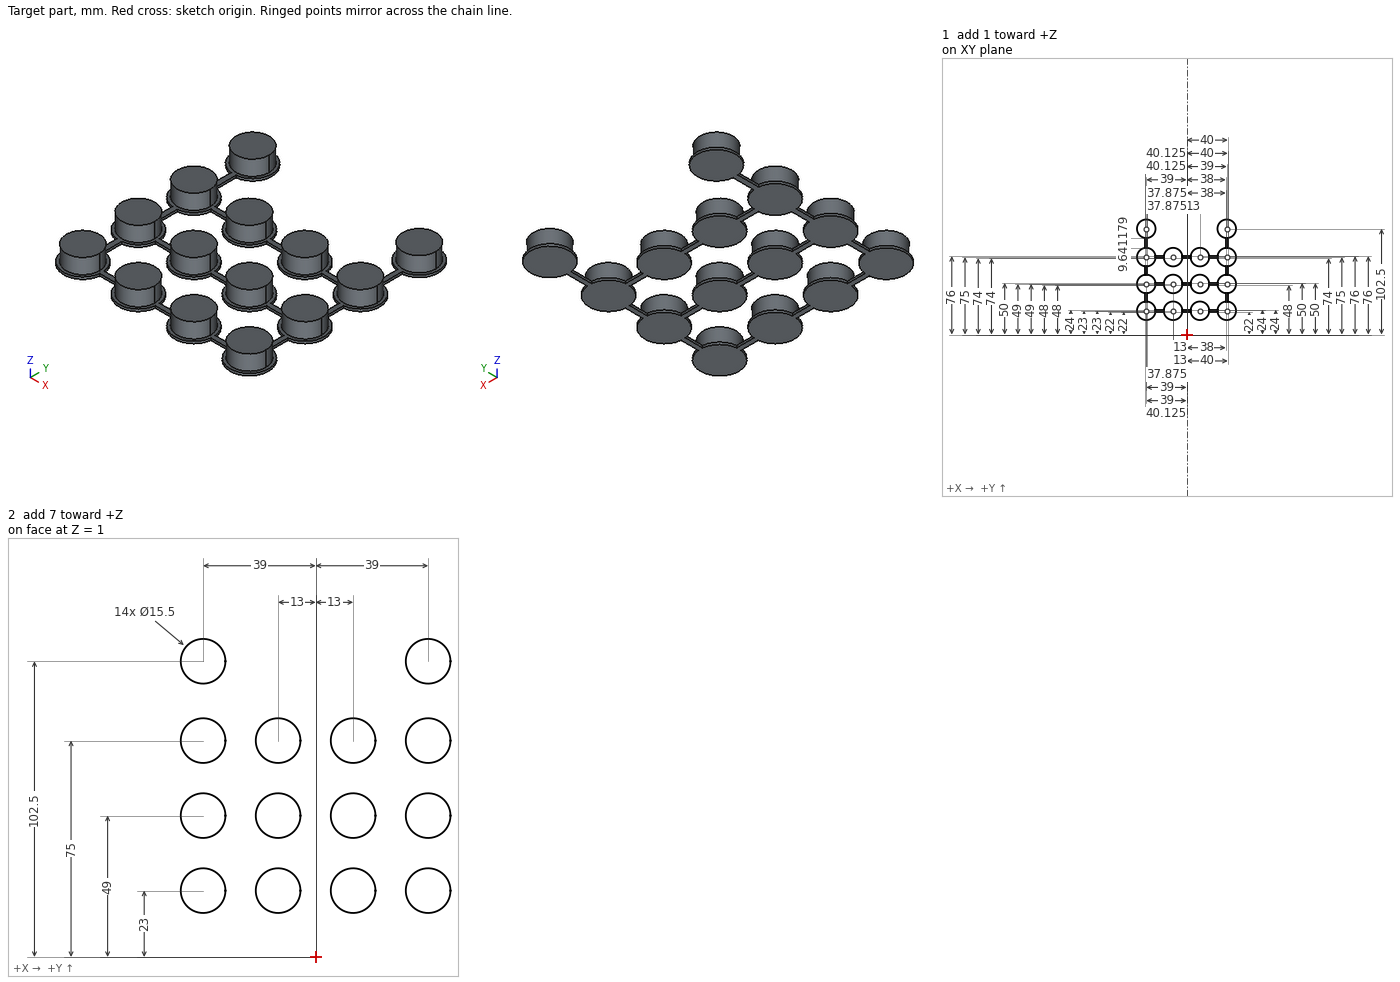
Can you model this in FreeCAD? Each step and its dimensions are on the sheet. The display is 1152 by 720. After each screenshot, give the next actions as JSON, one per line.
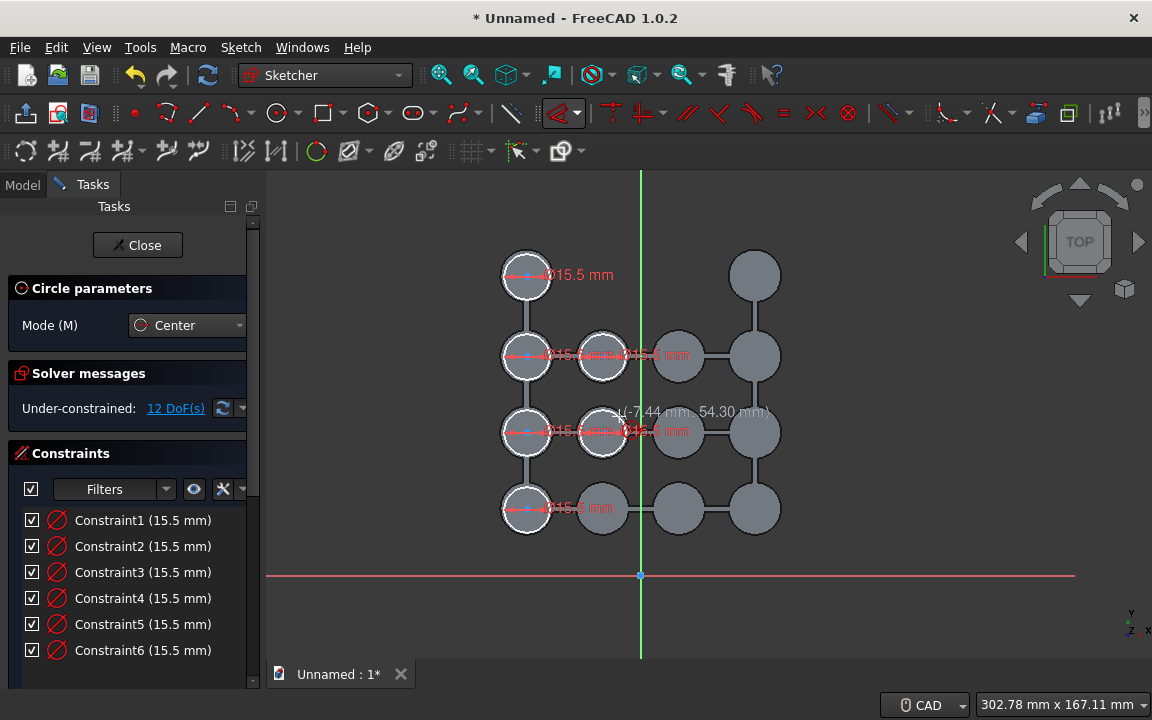
{"action": "left_click", "coordinate": [603, 509]}
{"action": "mouse_move", "coordinate": [619, 493]}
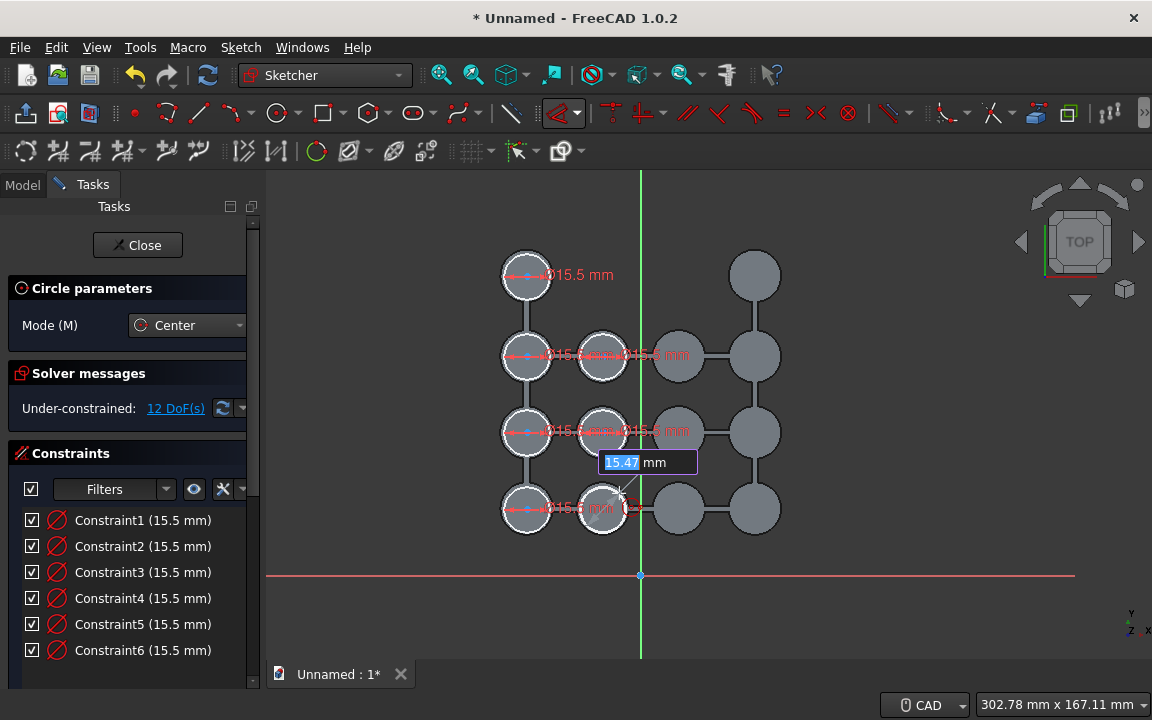
{"action": "type", "text": "15.5"}
{"action": "key", "text": "Return"}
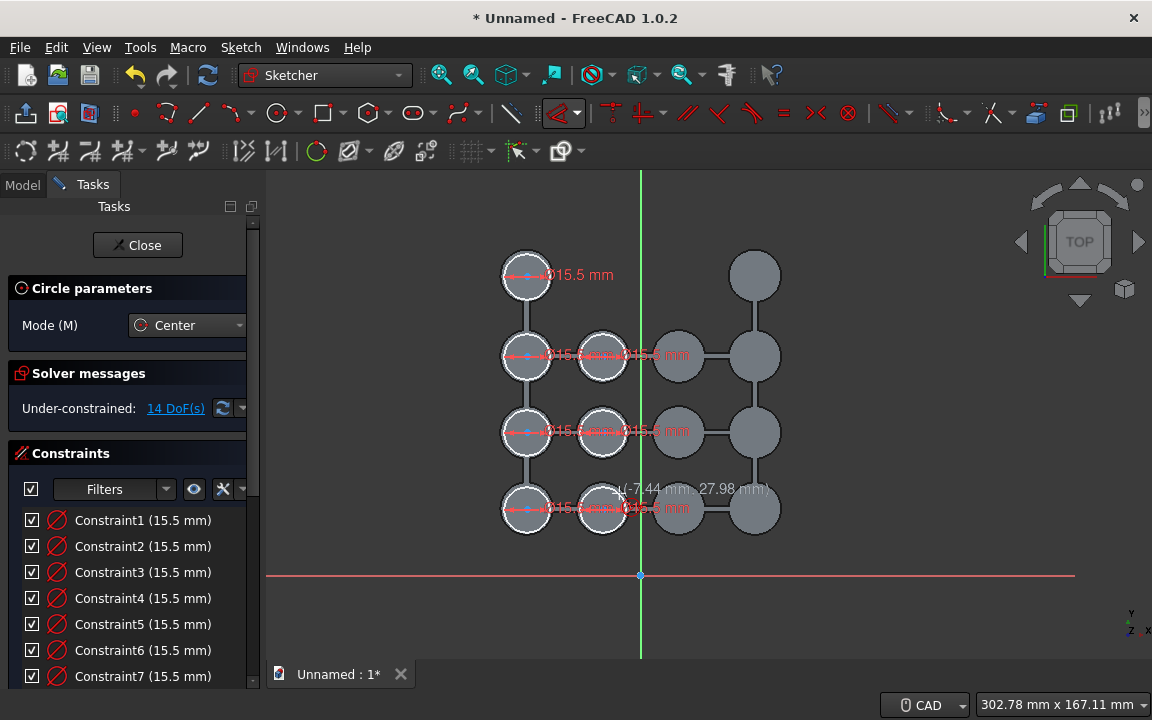
{"action": "left_click", "coordinate": [679, 356]}
{"action": "mouse_move", "coordinate": [695, 340]}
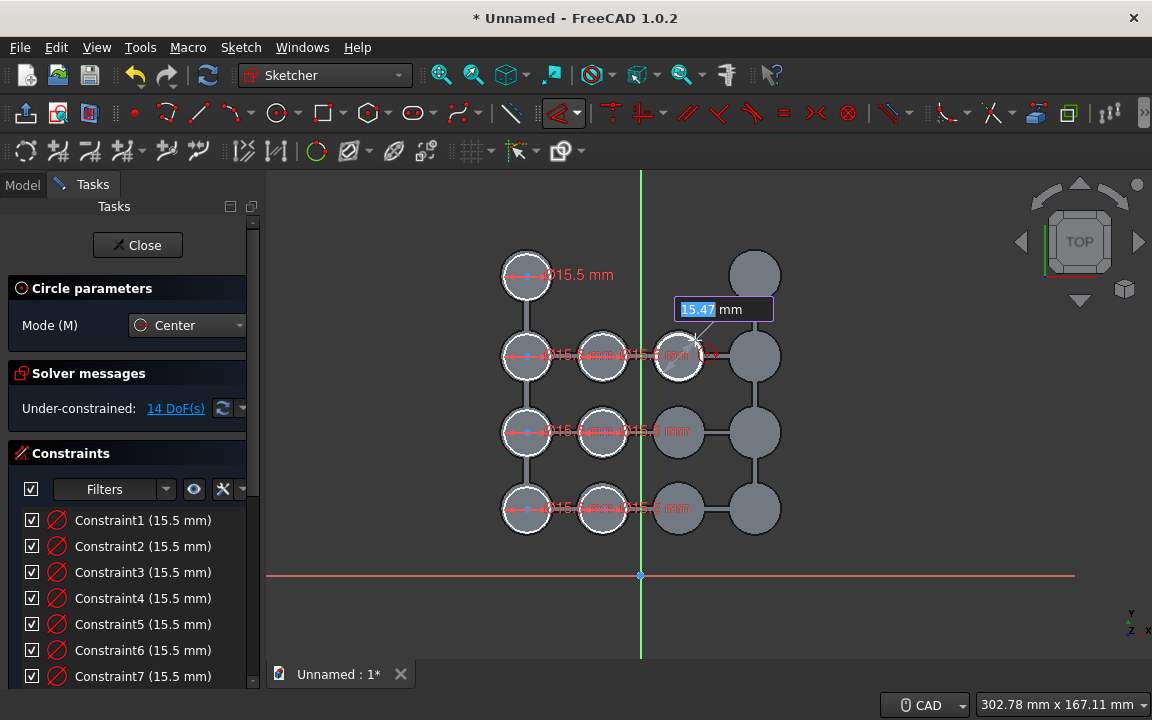
{"action": "type", "text": "15.5"}
{"action": "key", "text": "Return"}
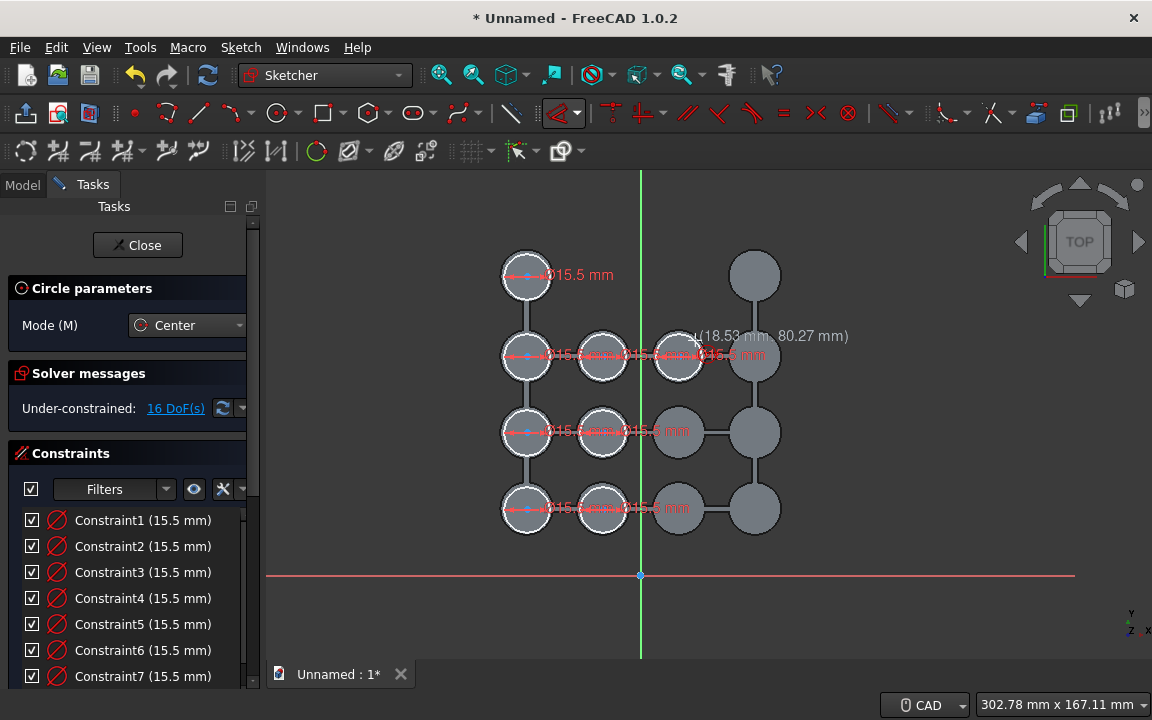
{"action": "left_click", "coordinate": [755, 276]}
{"action": "mouse_move", "coordinate": [771, 260]}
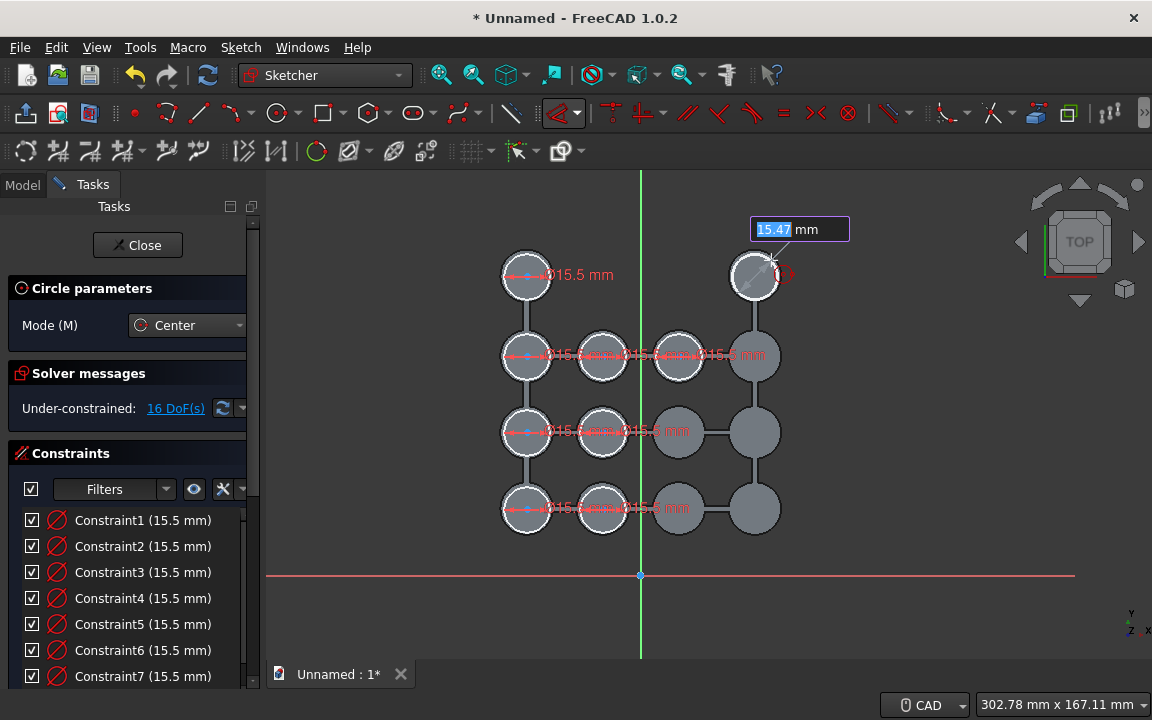
{"action": "type", "text": "15.5"}
{"action": "key", "text": "Return"}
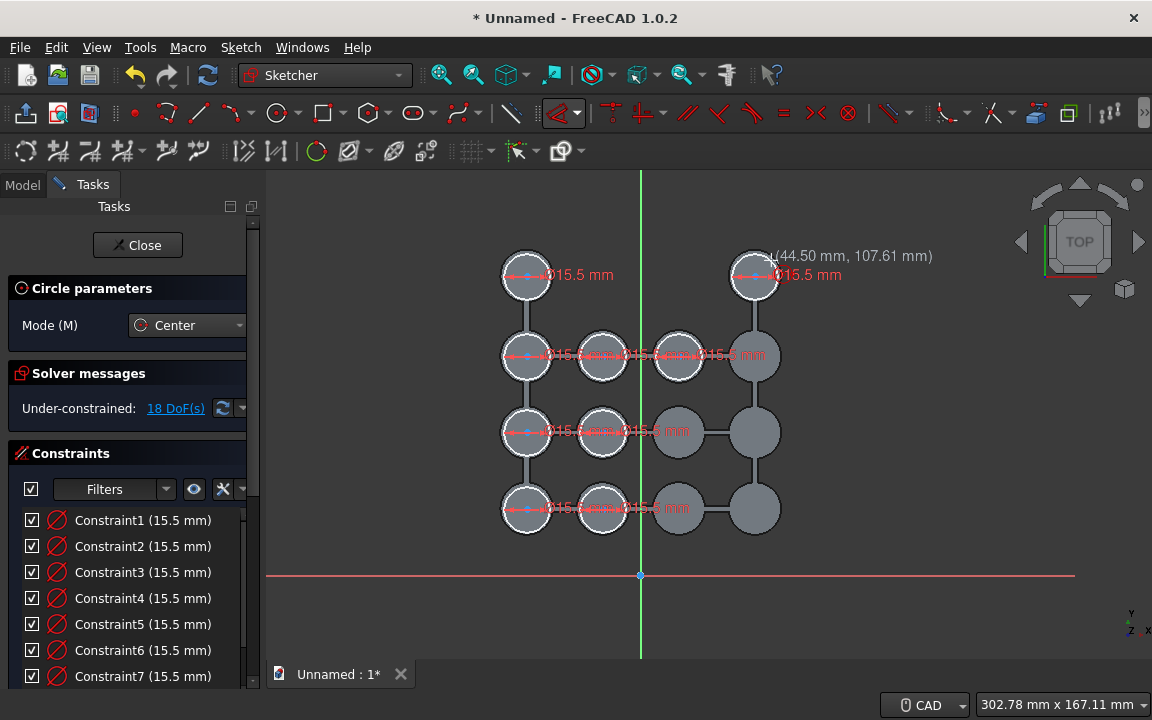
{"action": "left_click", "coordinate": [755, 509]}
{"action": "mouse_move", "coordinate": [771, 493]}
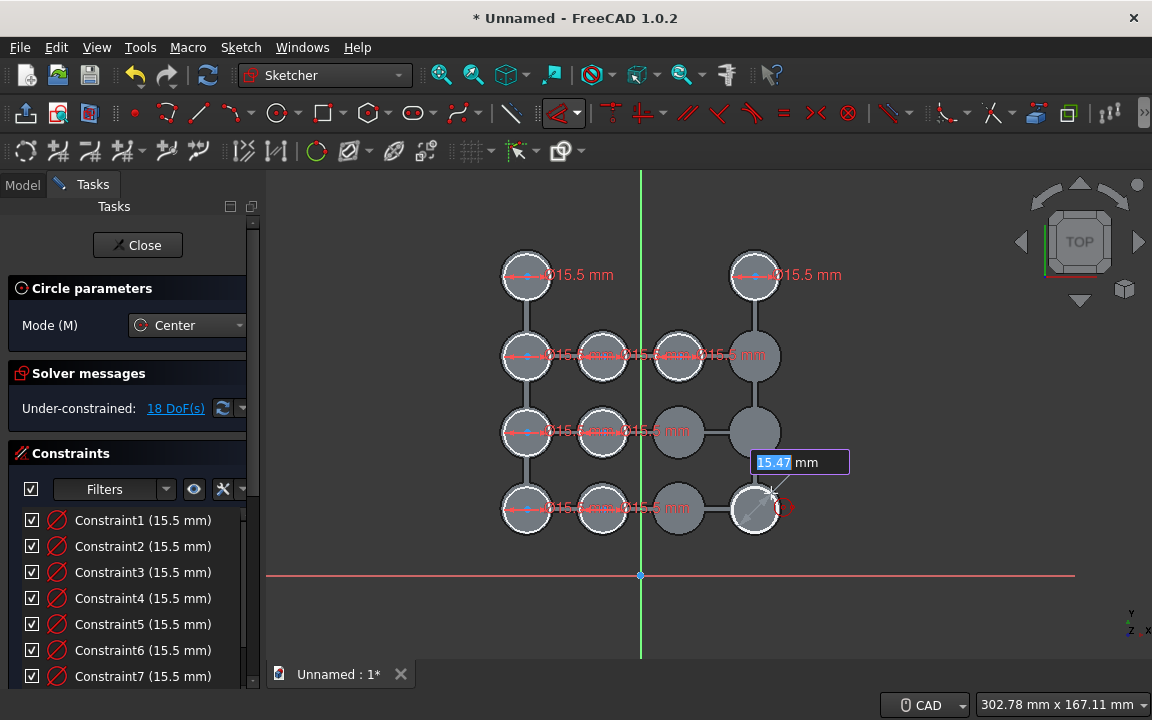
{"action": "type", "text": "15.5"}
{"action": "key", "text": "Return"}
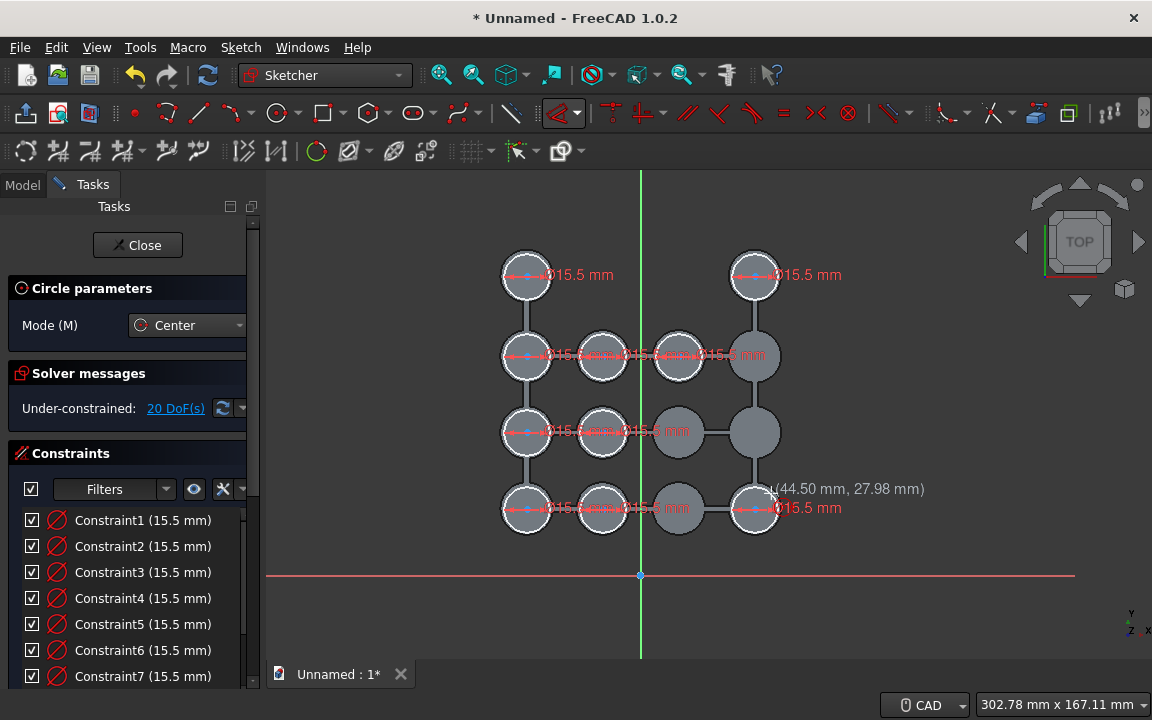
{"action": "left_click", "coordinate": [679, 509]}
{"action": "mouse_move", "coordinate": [695, 493]}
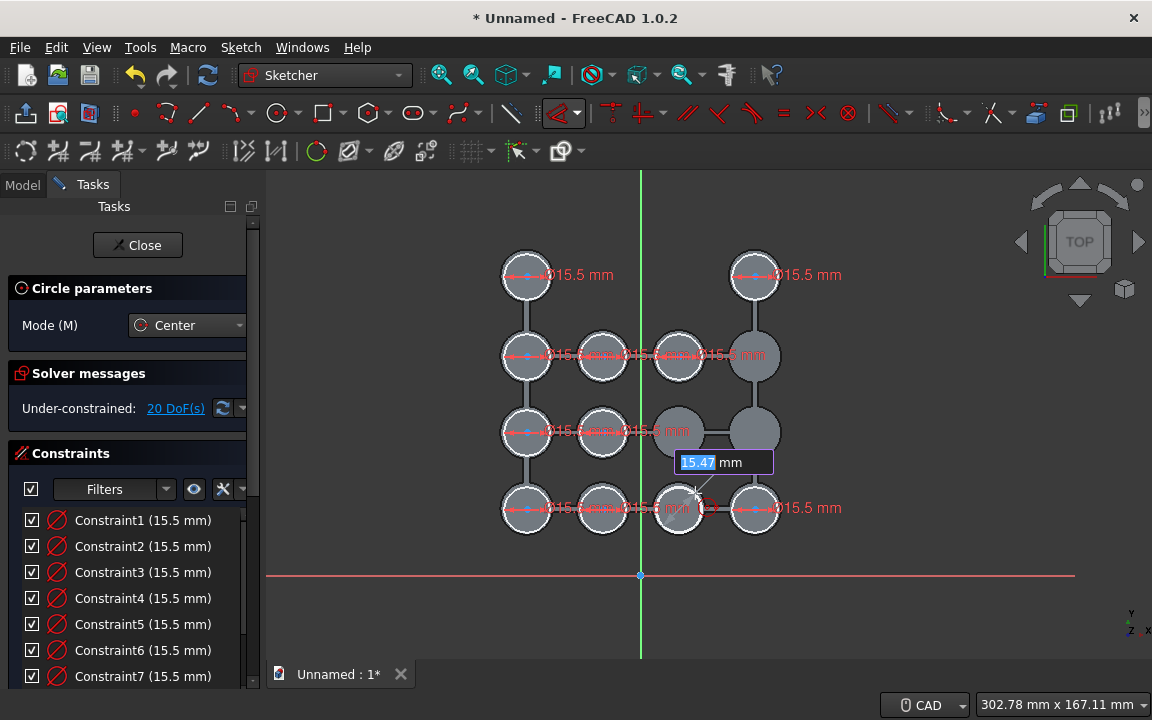
{"action": "type", "text": "15.5"}
{"action": "key", "text": "Return"}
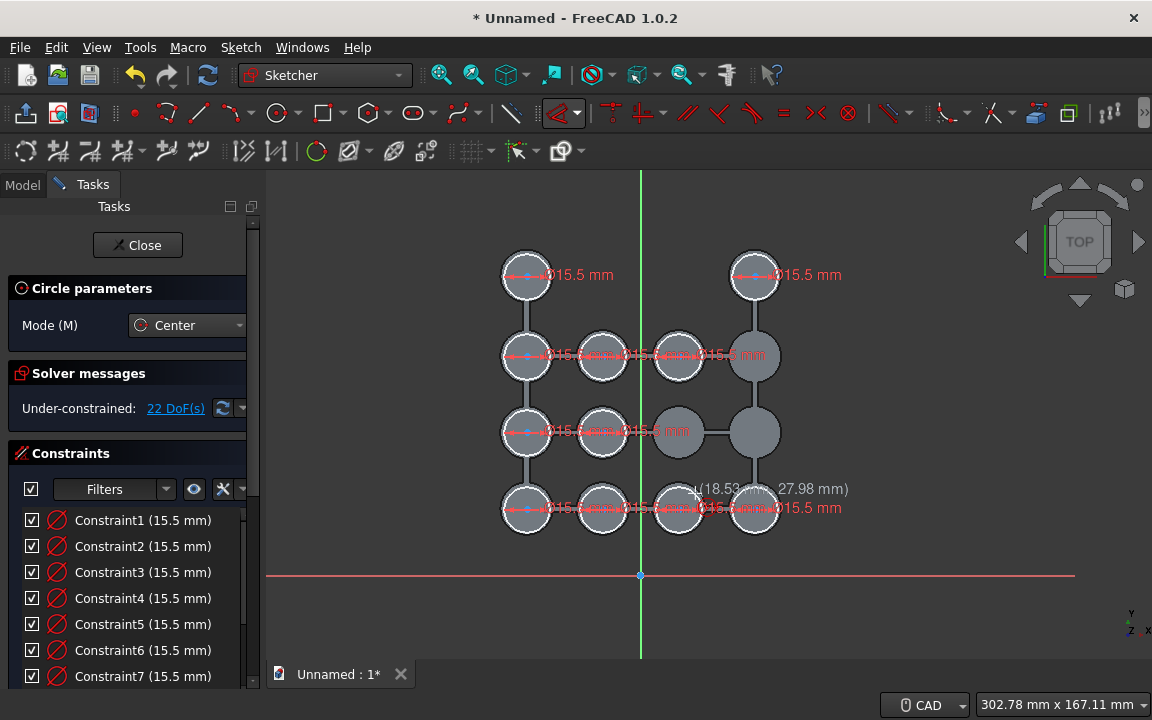
{"action": "left_click", "coordinate": [755, 432]}
{"action": "mouse_move", "coordinate": [771, 416]}